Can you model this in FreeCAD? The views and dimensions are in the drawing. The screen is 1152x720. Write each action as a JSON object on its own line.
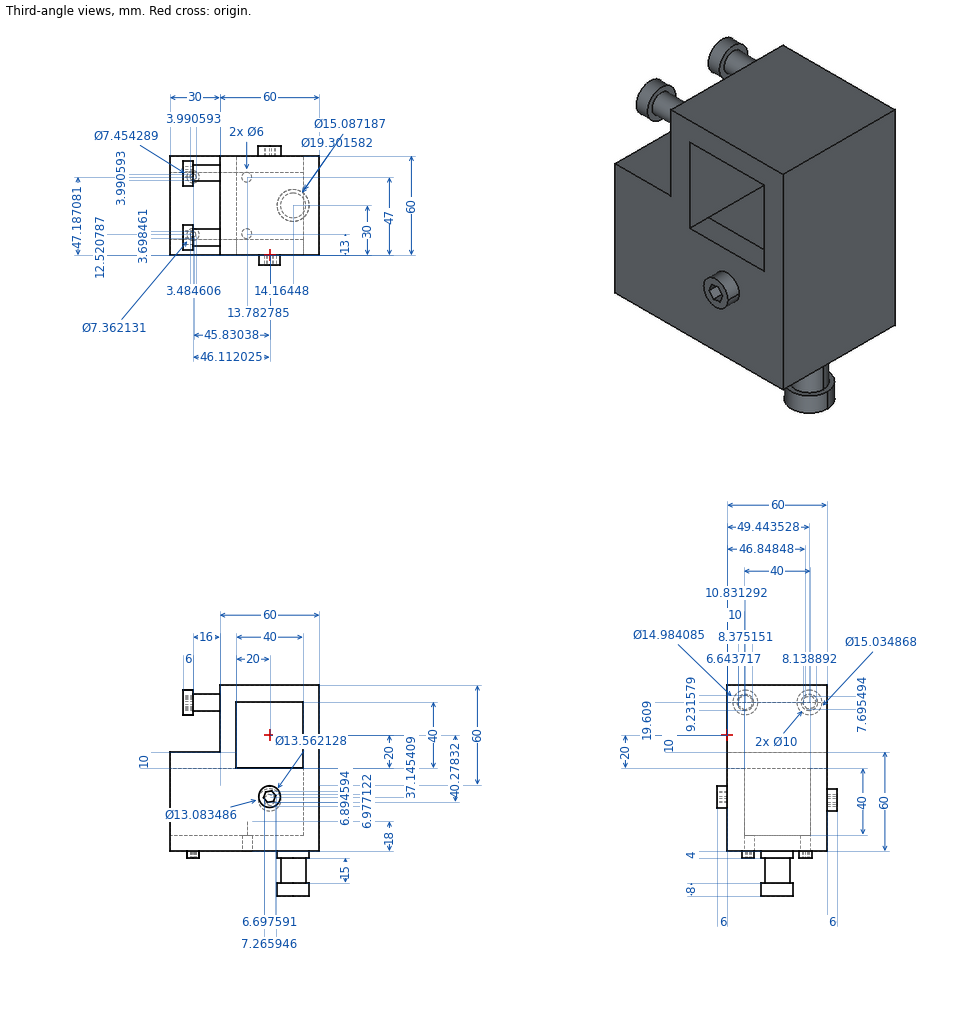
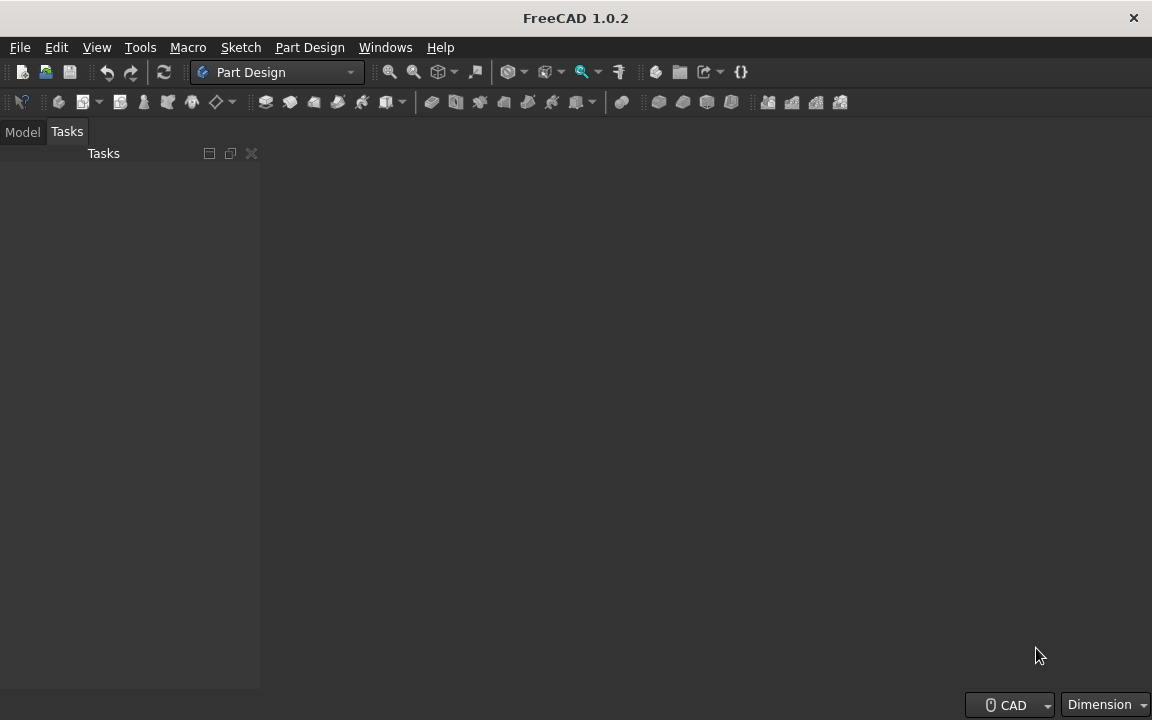
{"action": "left_click", "coordinate": [22, 72]}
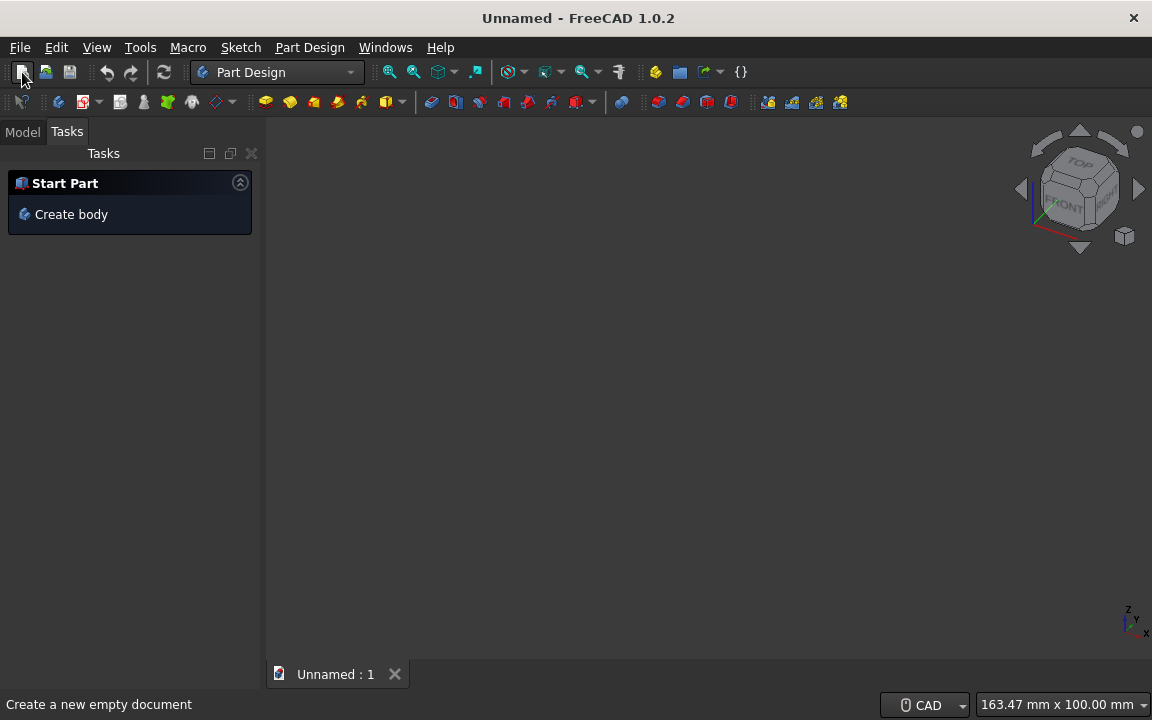
{"action": "left_click", "coordinate": [84, 102]}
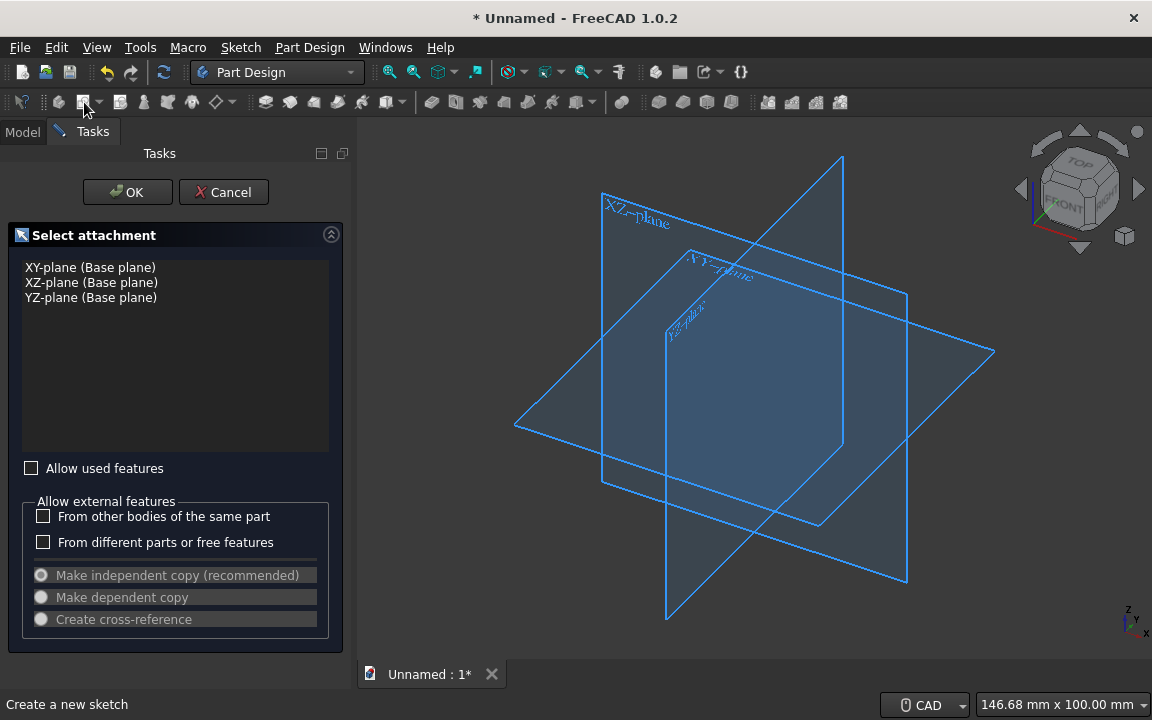
{"action": "left_click", "coordinate": [82, 282]}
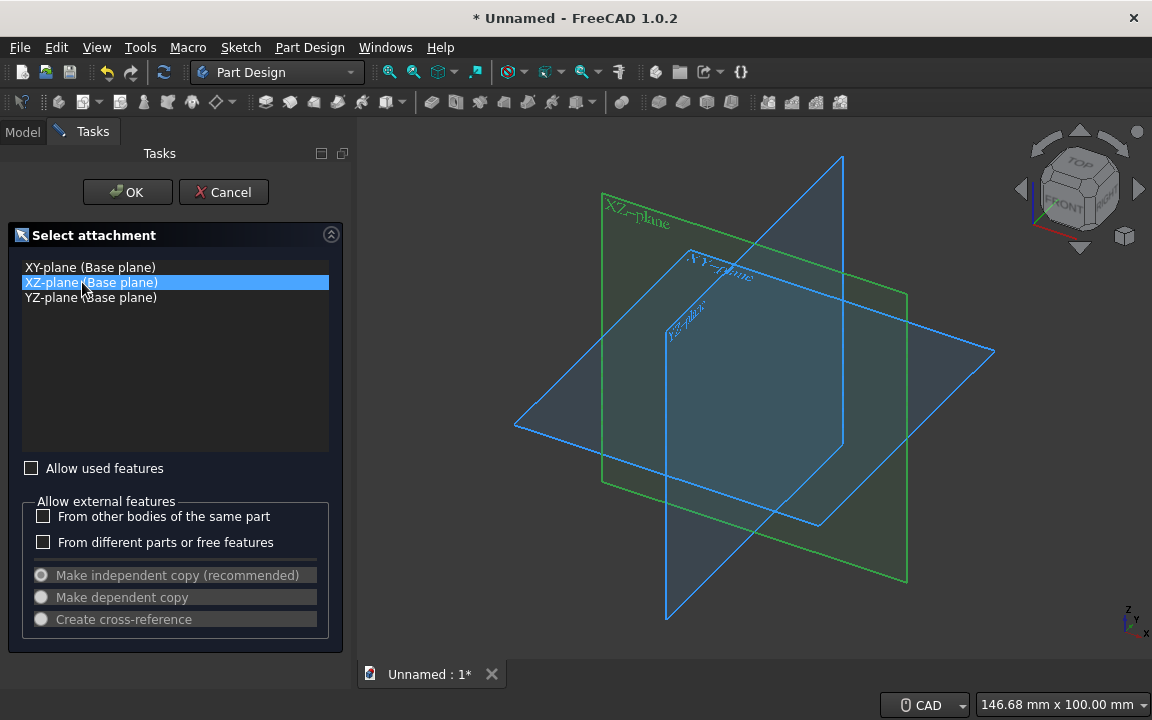
{"action": "left_click", "coordinate": [128, 192]}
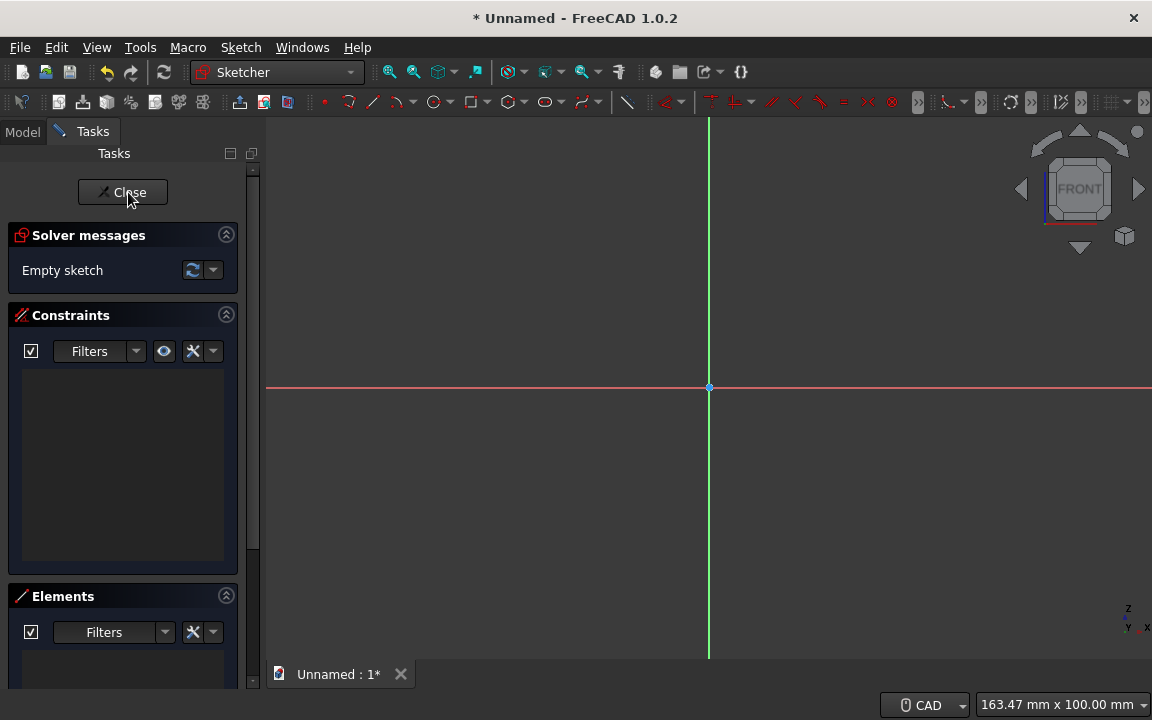
{"action": "left_click", "coordinate": [490, 102]}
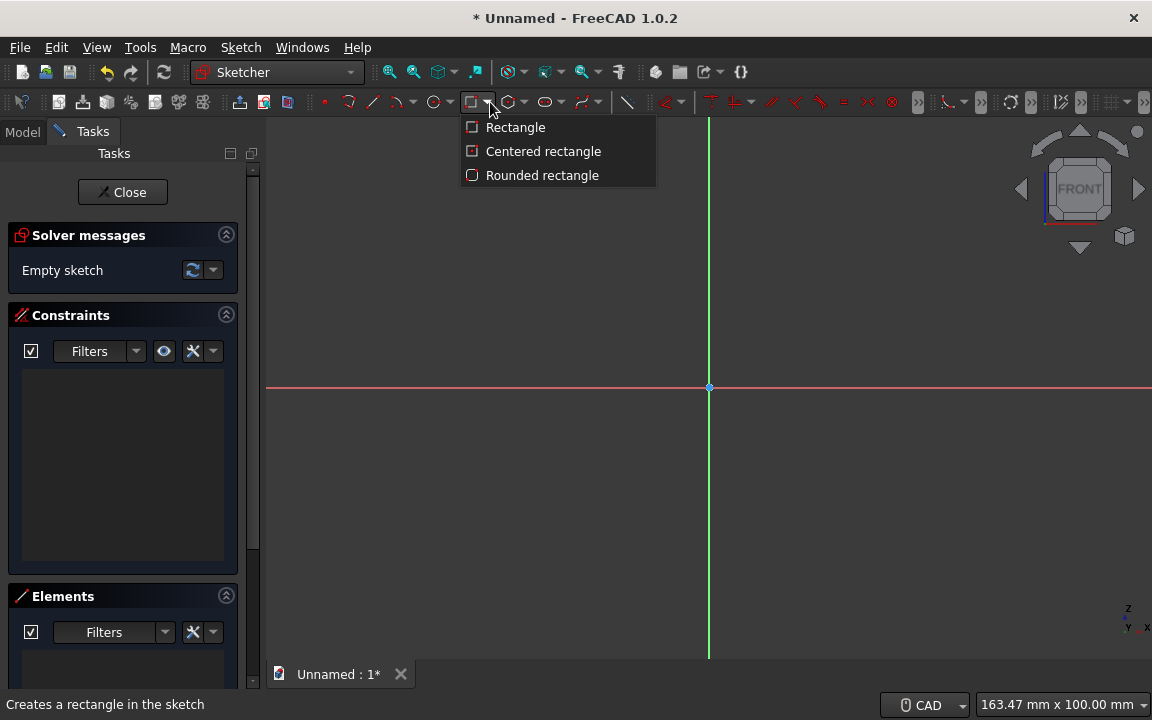
{"action": "left_click", "coordinate": [558, 151]}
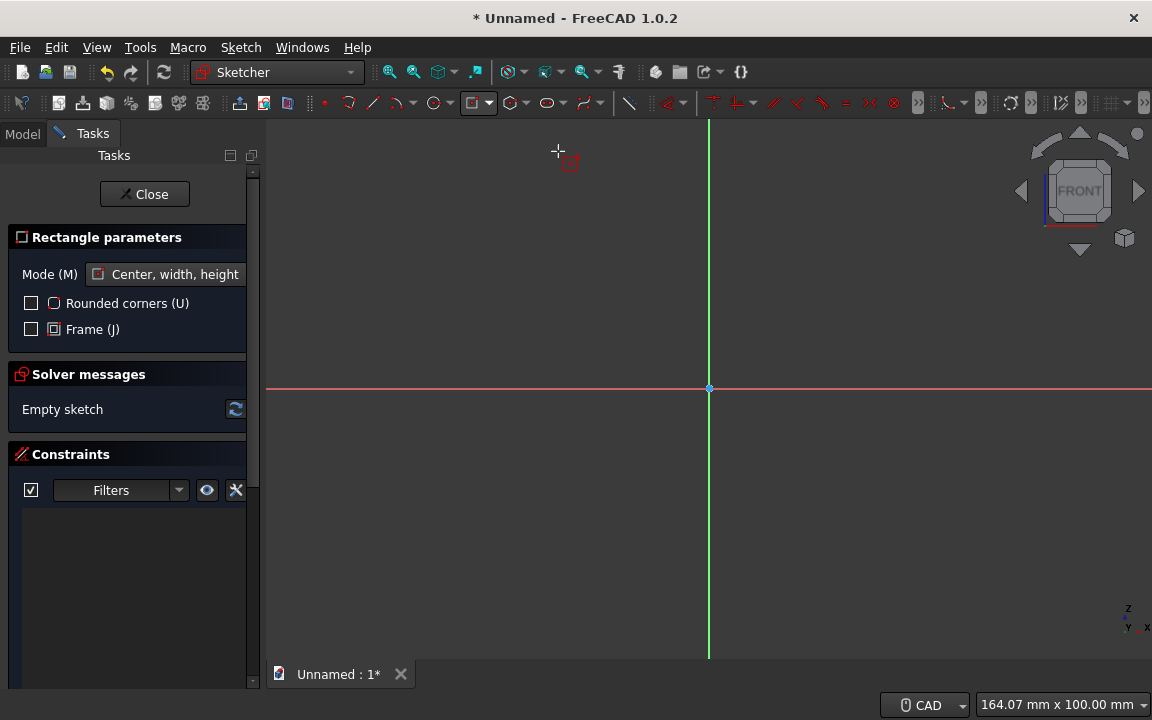
{"action": "left_click", "coordinate": [709, 389]}
{"action": "left_click", "coordinate": [871, 227]}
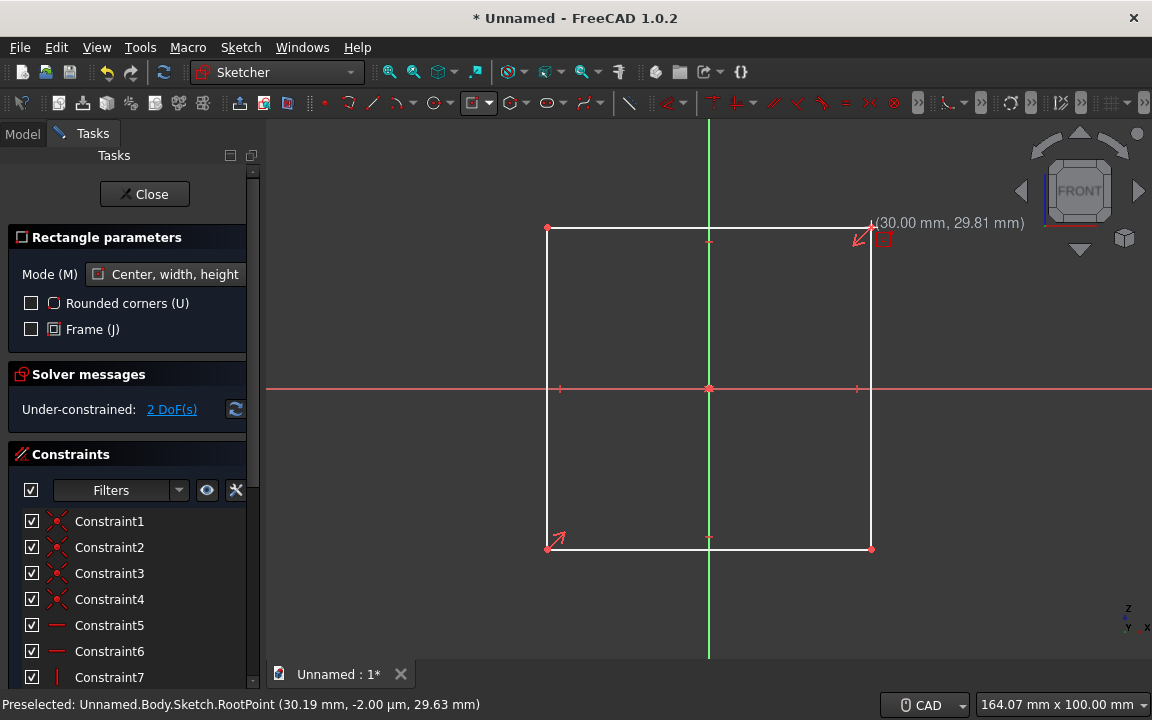
{"action": "left_click", "coordinate": [709, 389]}
{"action": "left_click", "coordinate": [817, 281]}
{"action": "key", "text": "Escape"}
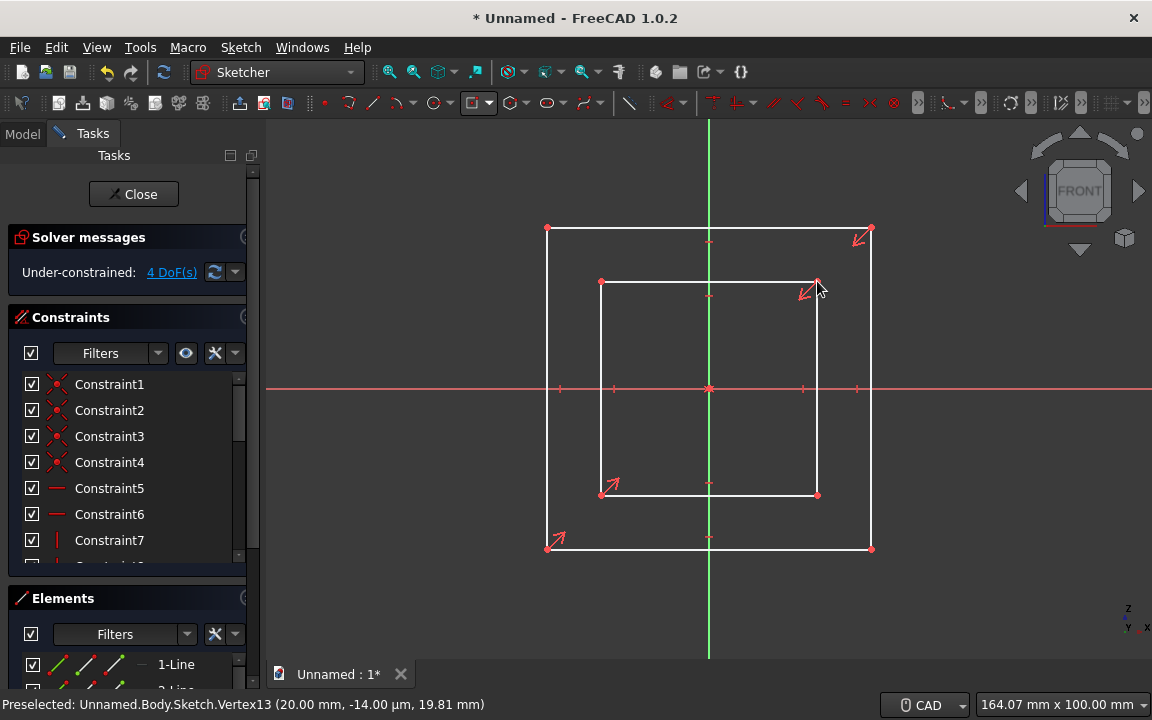
{"action": "left_click", "coordinate": [668, 104]}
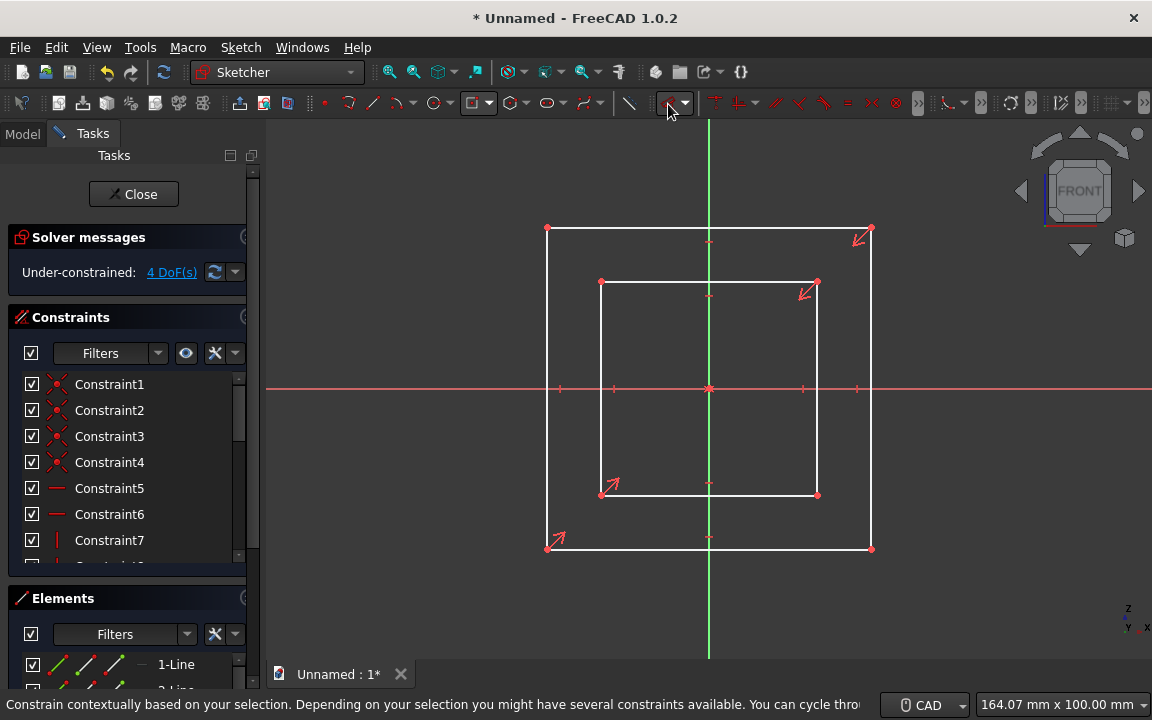
{"action": "left_click", "coordinate": [644, 550]}
{"action": "left_click", "coordinate": [634, 584]}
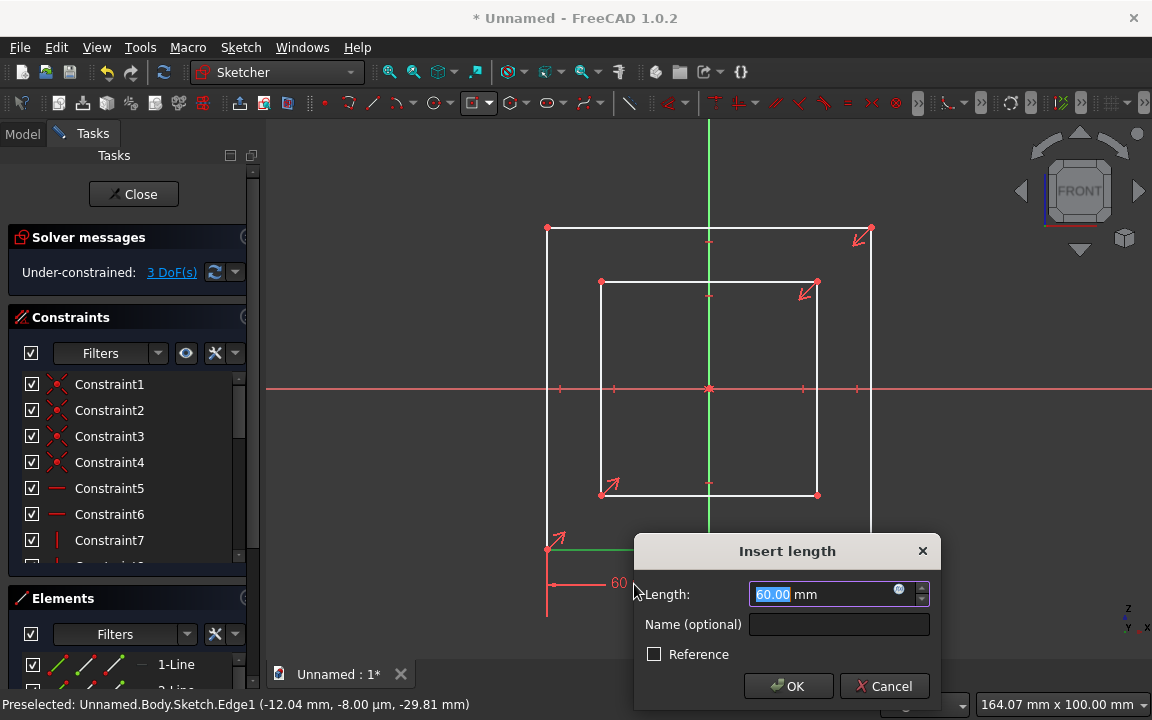
{"action": "type", "text": "60"}
{"action": "key", "text": "Return"}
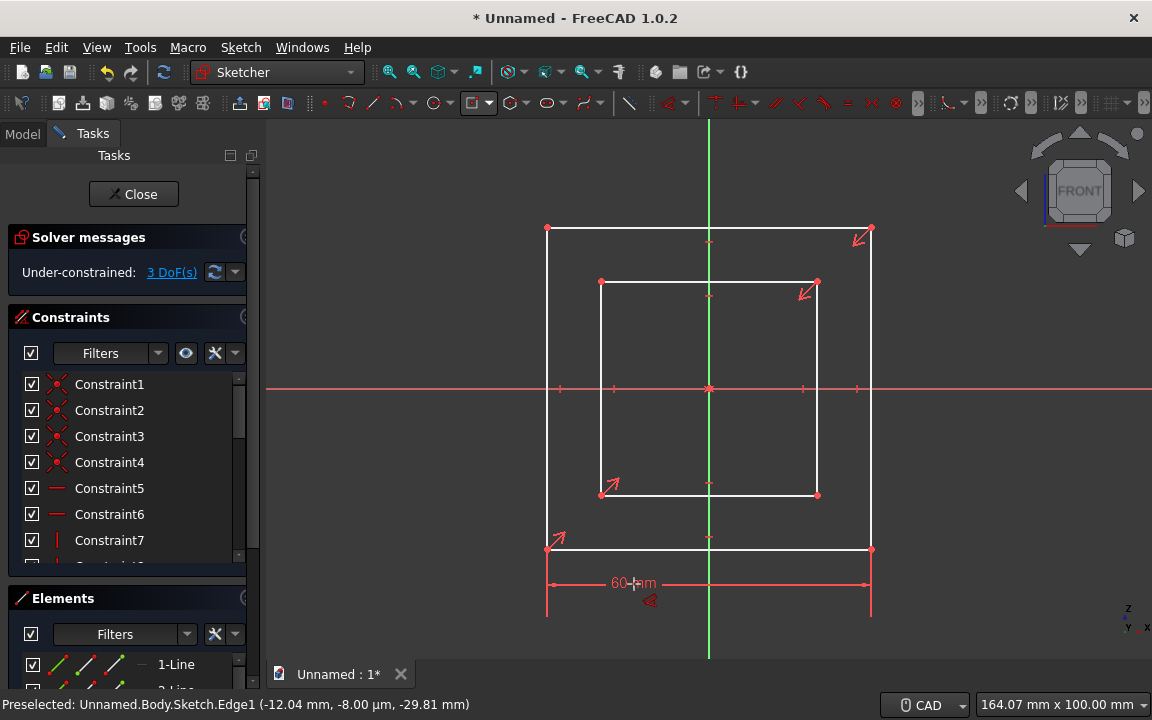
{"action": "left_click", "coordinate": [871, 453]}
{"action": "left_click", "coordinate": [905, 315]}